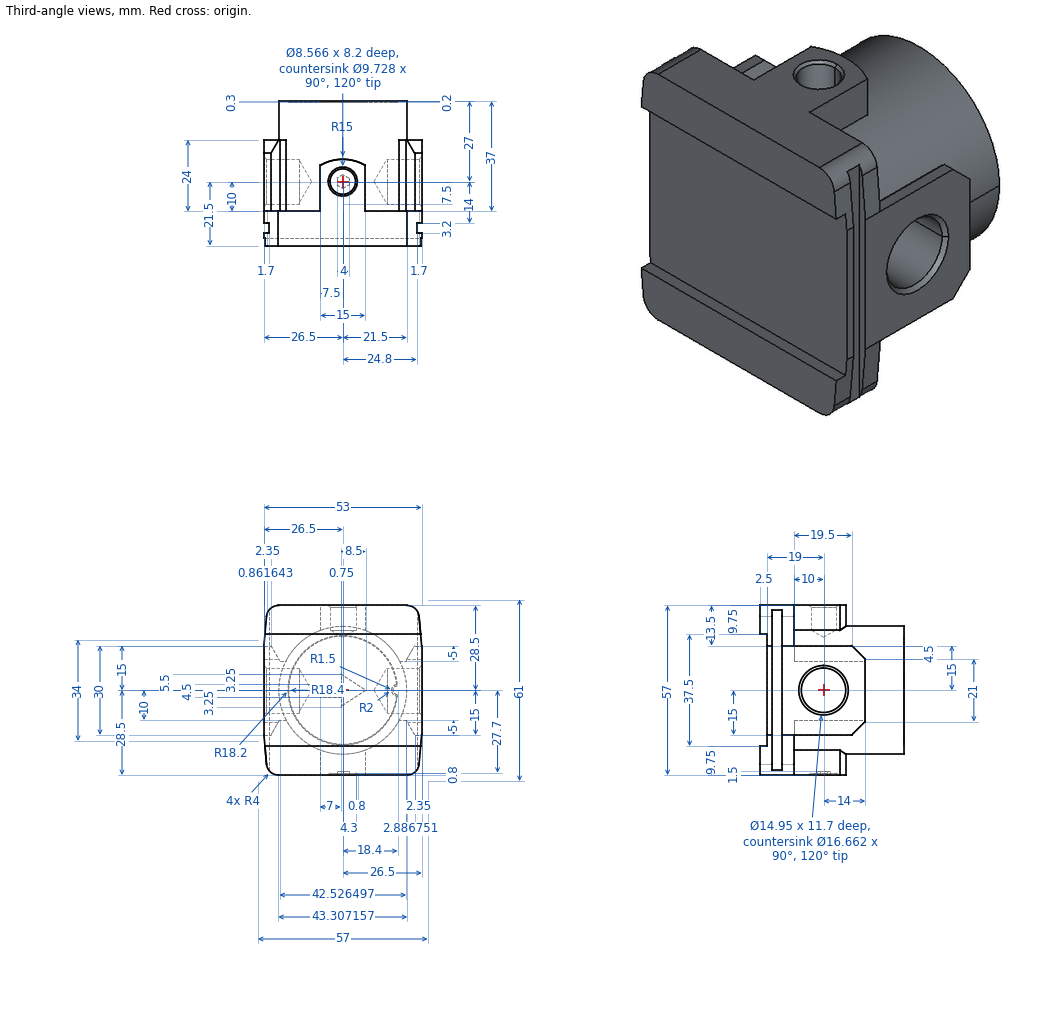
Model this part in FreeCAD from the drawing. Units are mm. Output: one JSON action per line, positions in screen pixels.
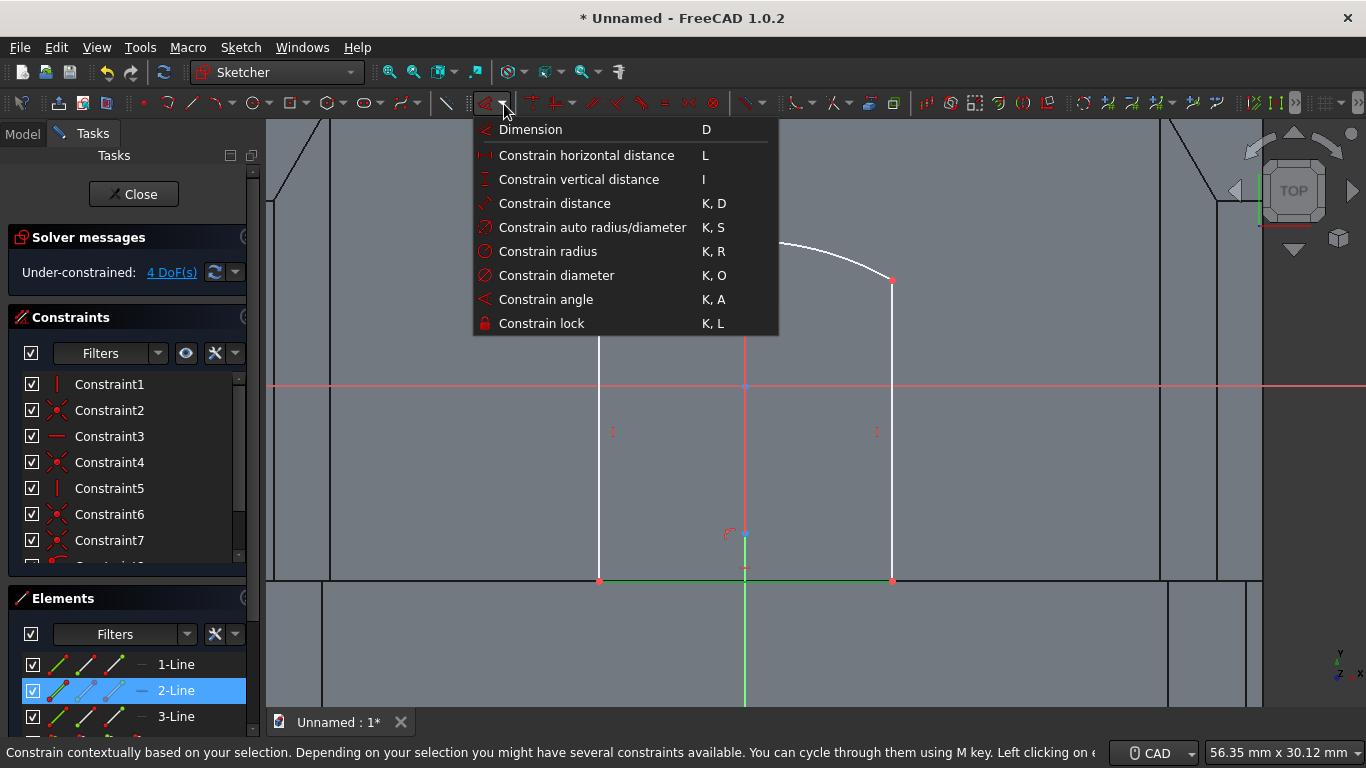
{"action": "left_click", "coordinate": [626, 155]}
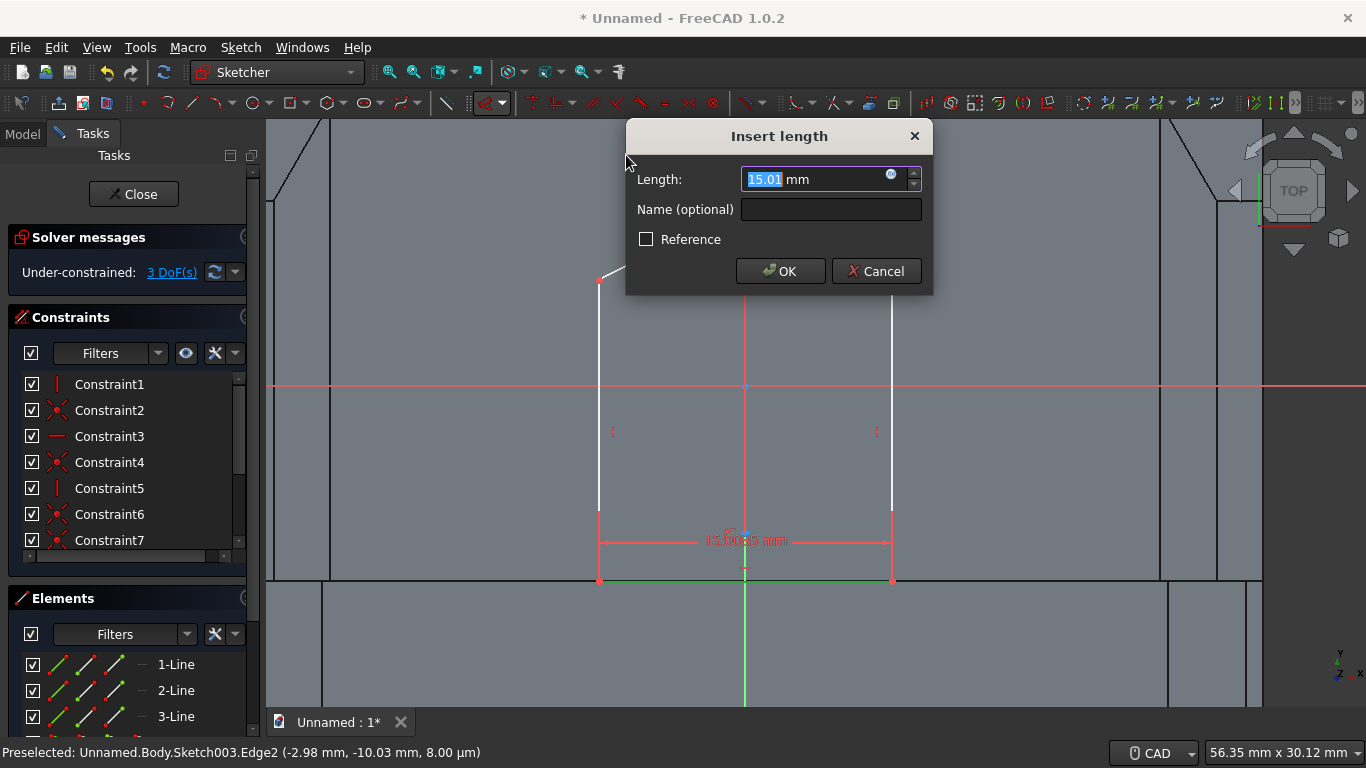
{"action": "type", "text": "15"}
{"action": "key", "text": "Return"}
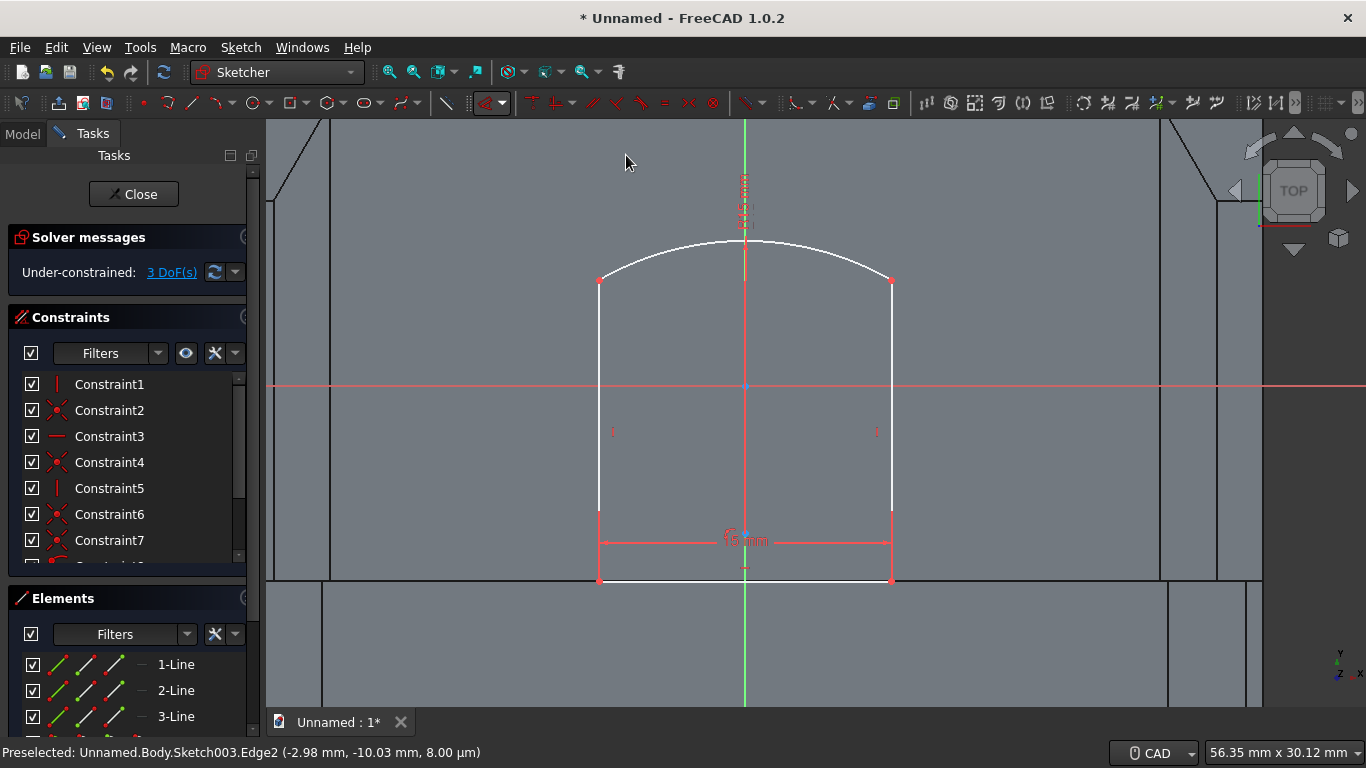
{"action": "left_click", "coordinate": [599, 582]}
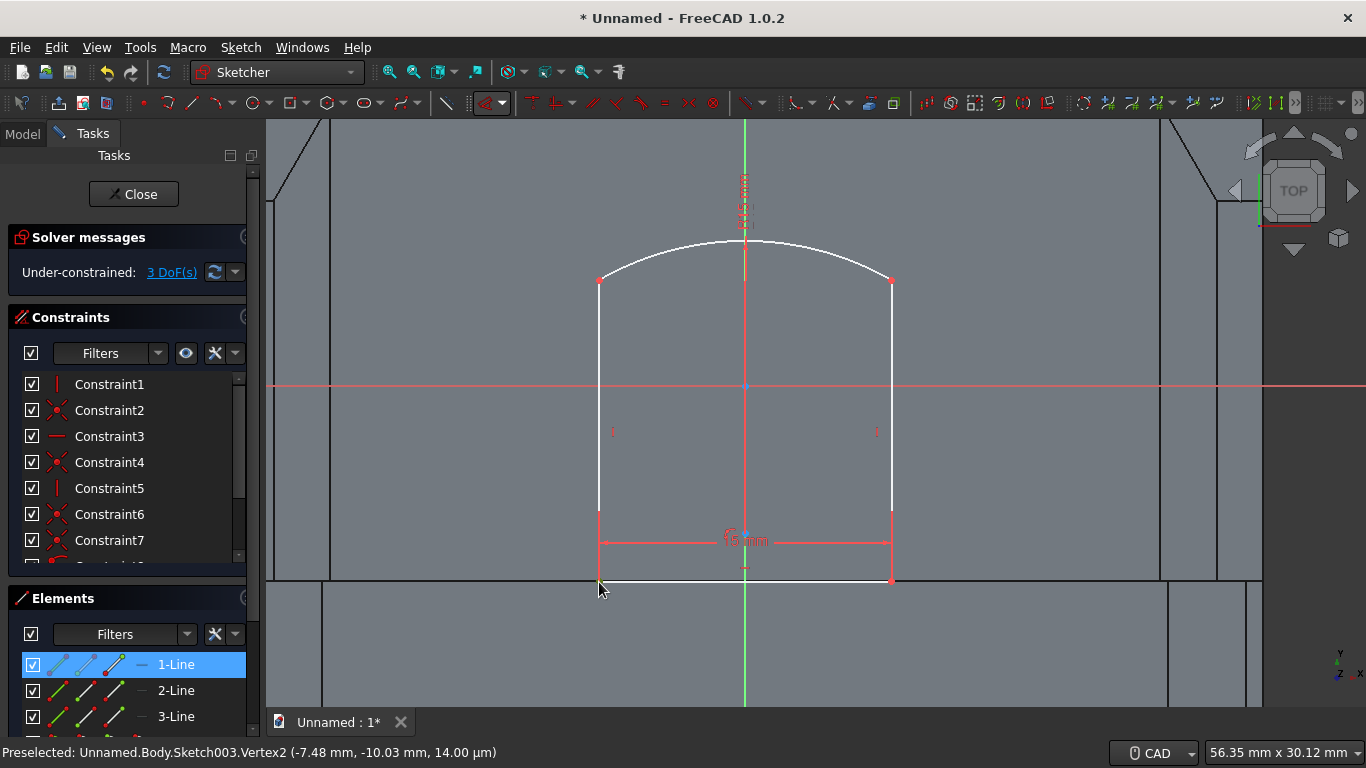
{"action": "key", "text": "i"}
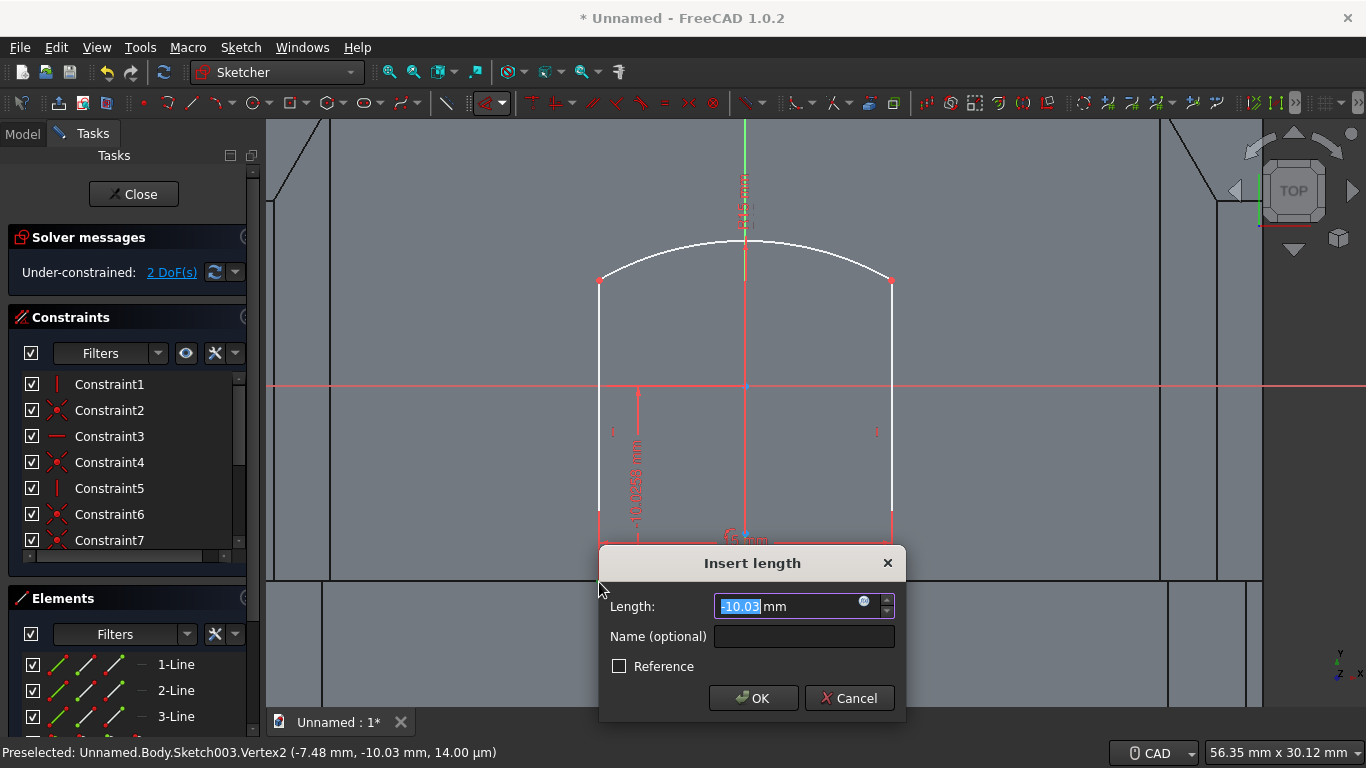
{"action": "type", "text": "-10"}
{"action": "key", "text": "Return"}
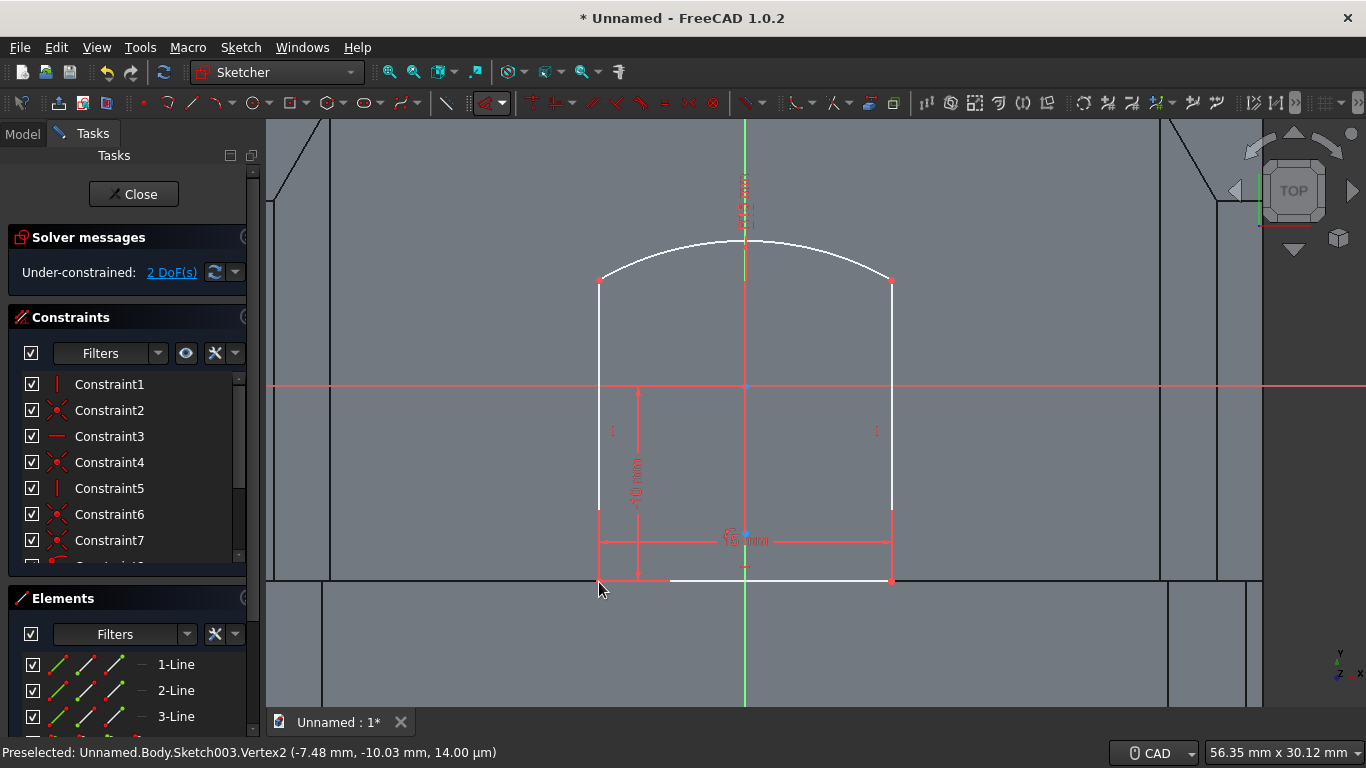
{"action": "left_click", "coordinate": [599, 280]}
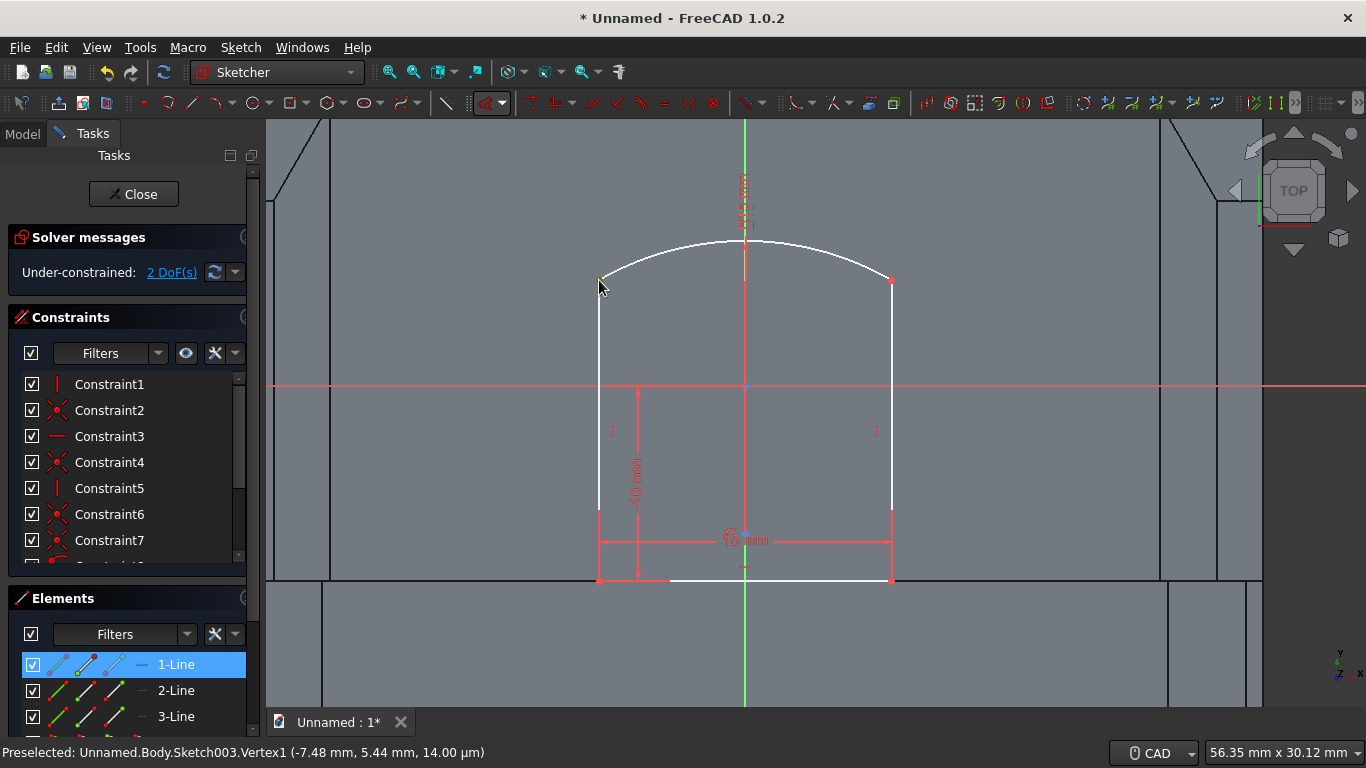
{"action": "key", "text": "l"}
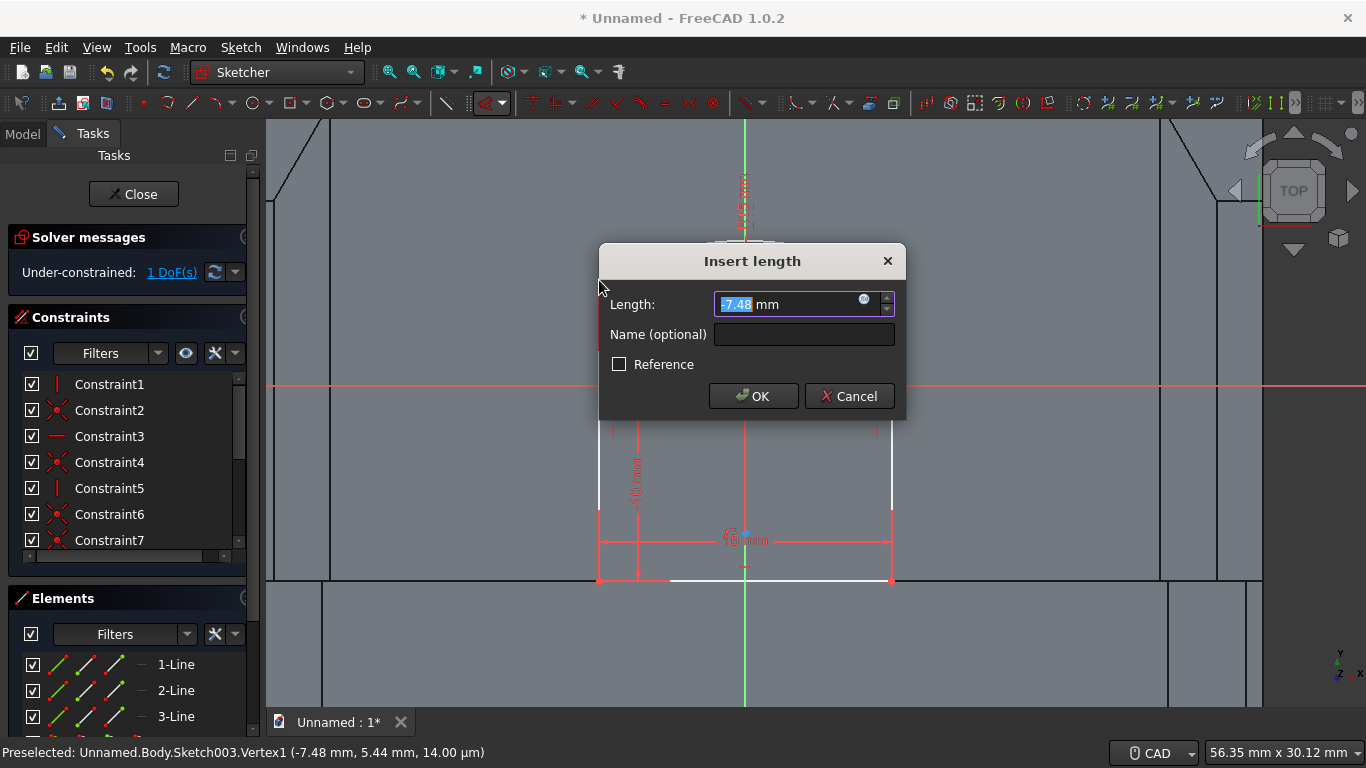
{"action": "type", "text": "-7.5"}
{"action": "key", "text": "Return"}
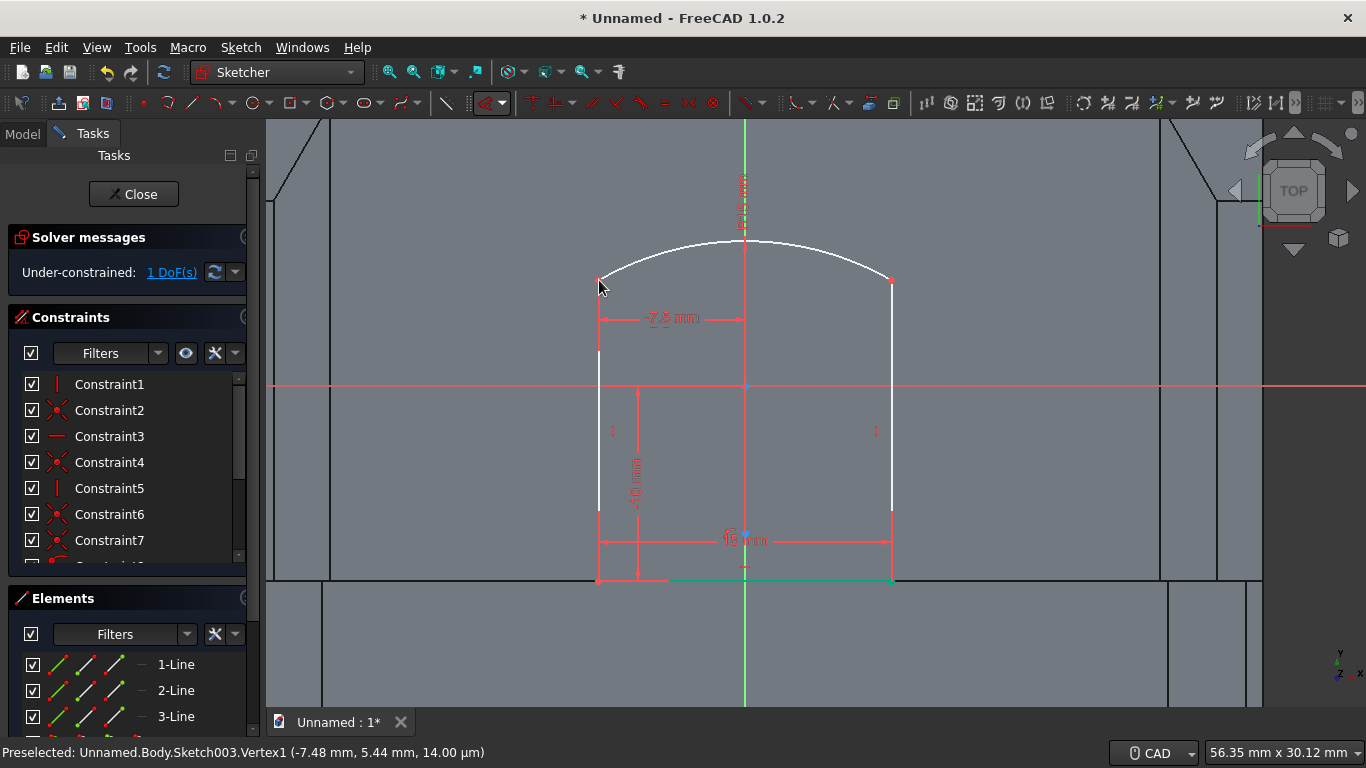
{"action": "left_click", "coordinate": [745, 534]}